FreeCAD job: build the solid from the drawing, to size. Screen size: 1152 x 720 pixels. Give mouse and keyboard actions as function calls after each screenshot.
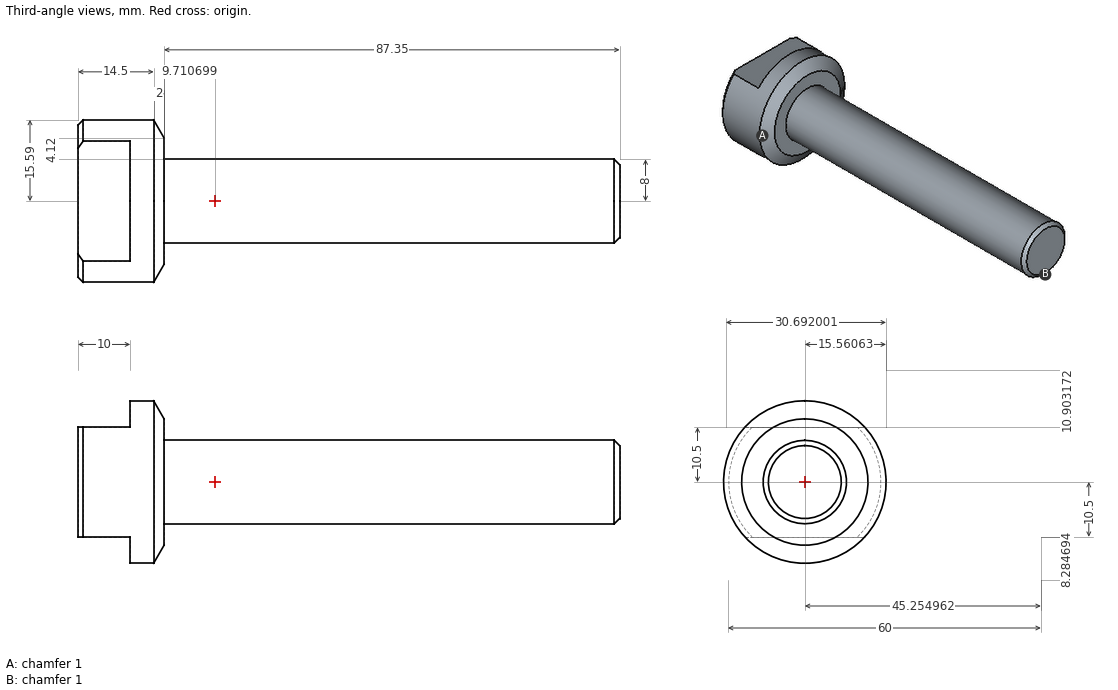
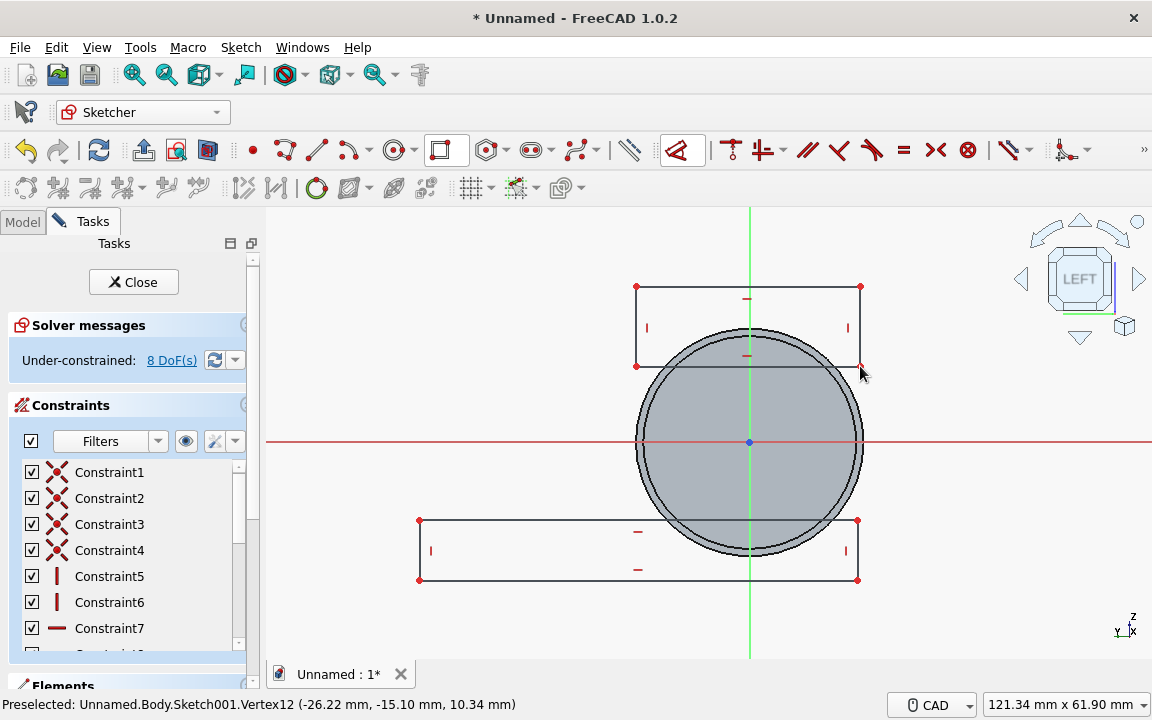
click(551, 581)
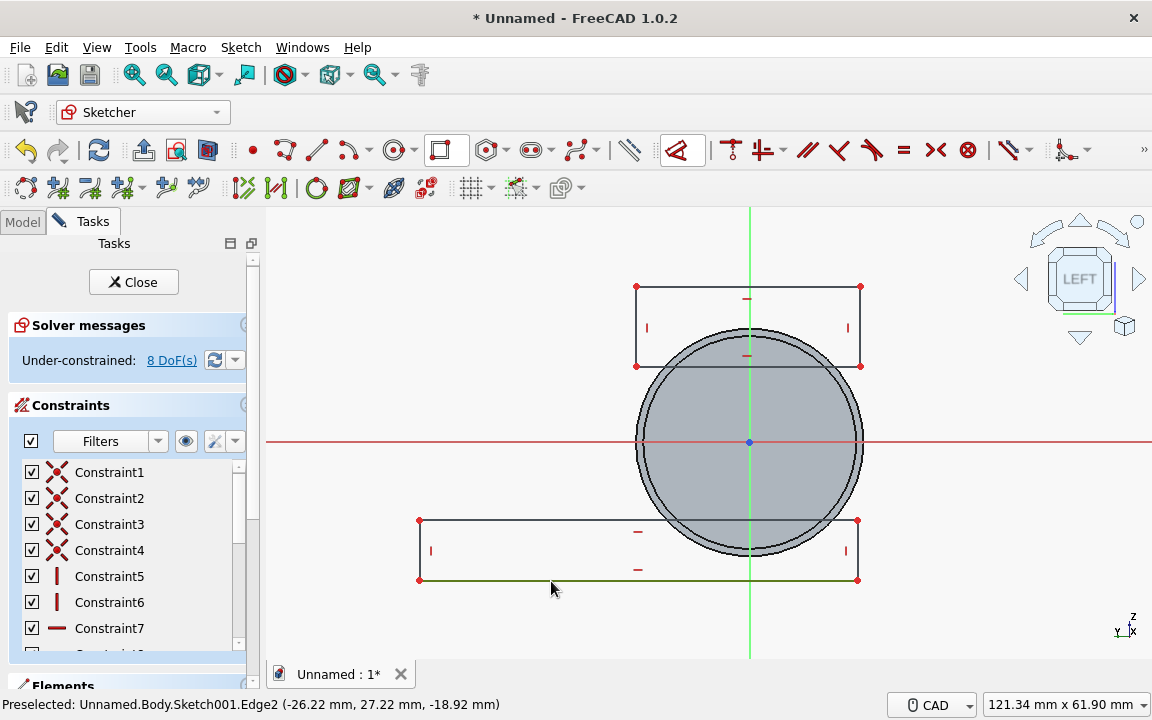
click(700, 150)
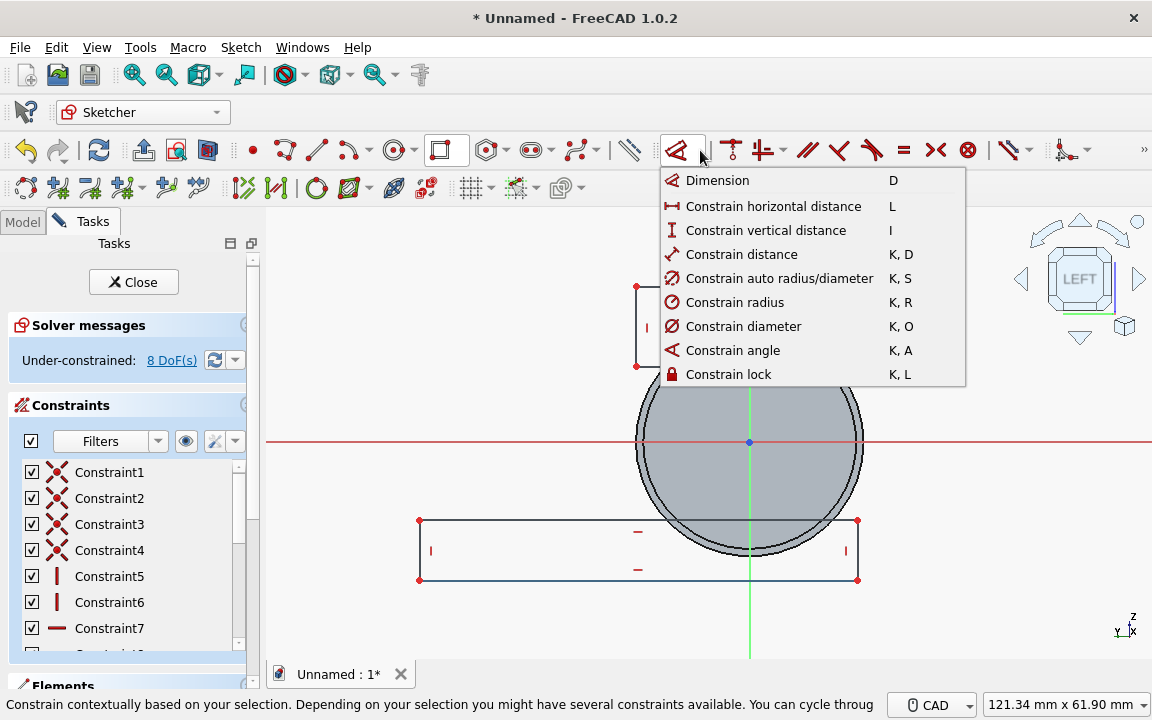
click(813, 206)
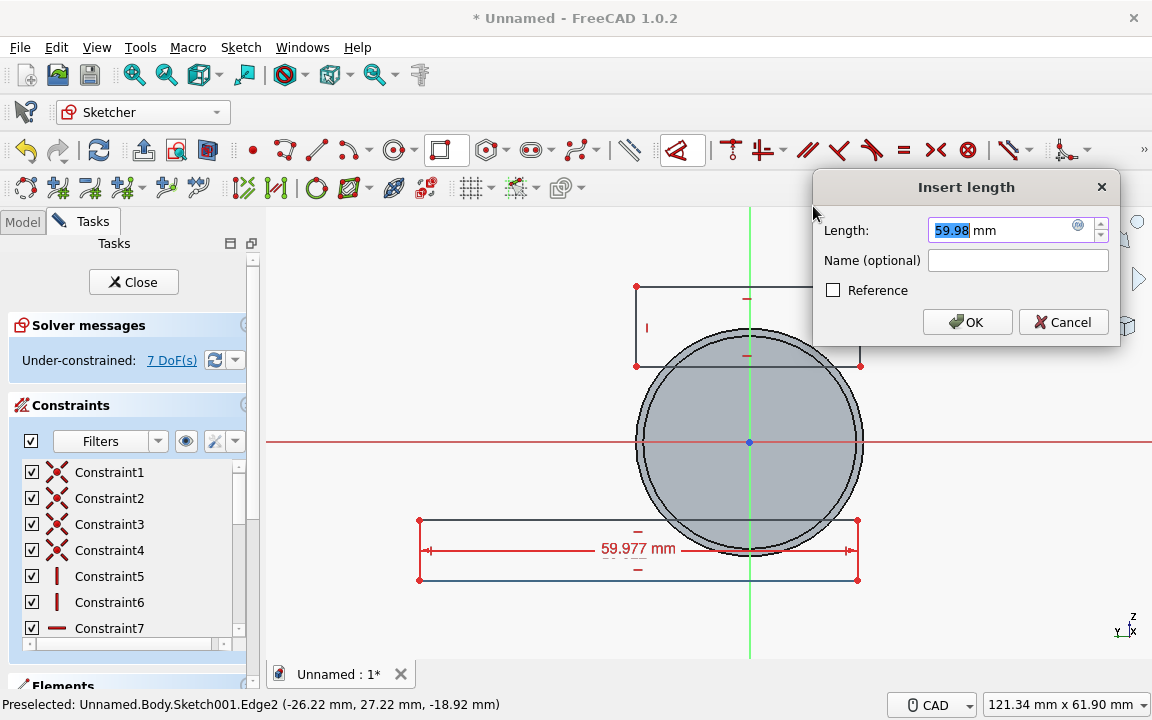
text(60)
key(Return)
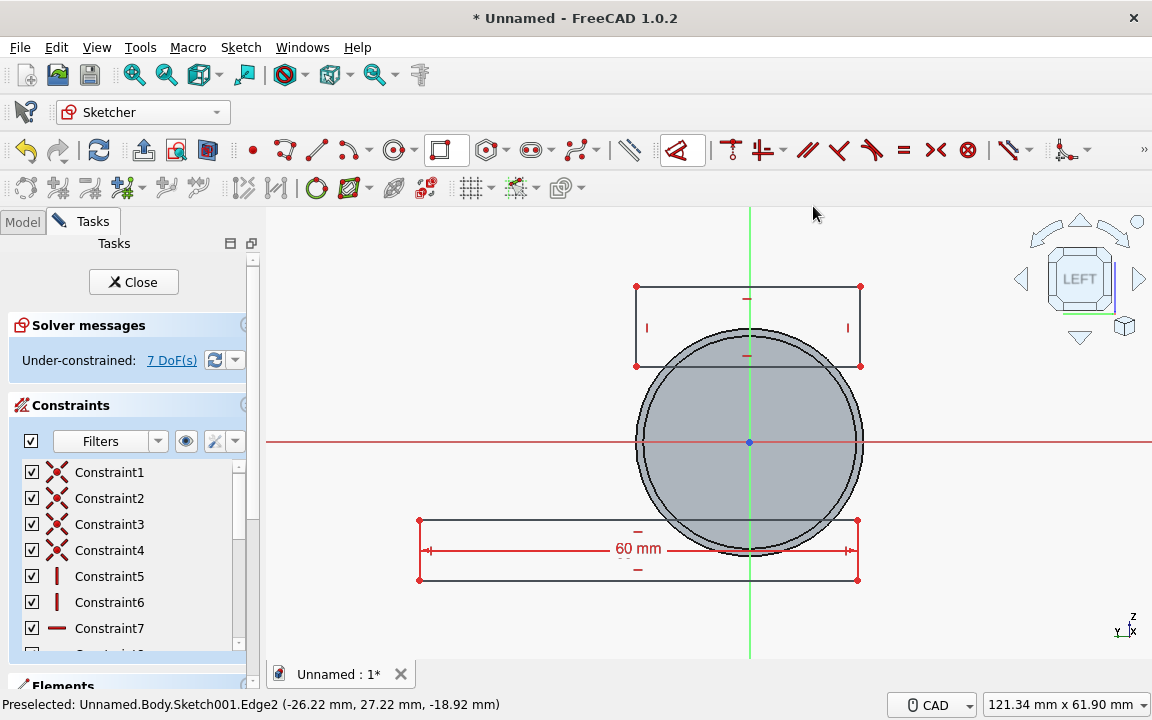
click(420, 520)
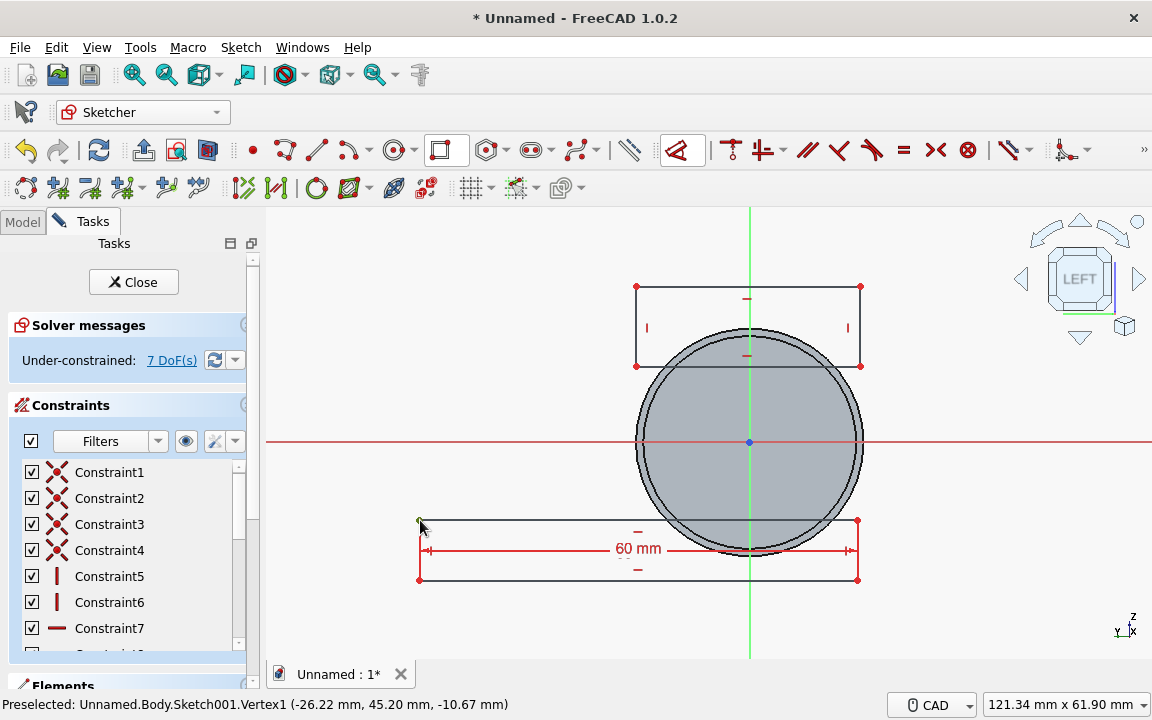
key(i)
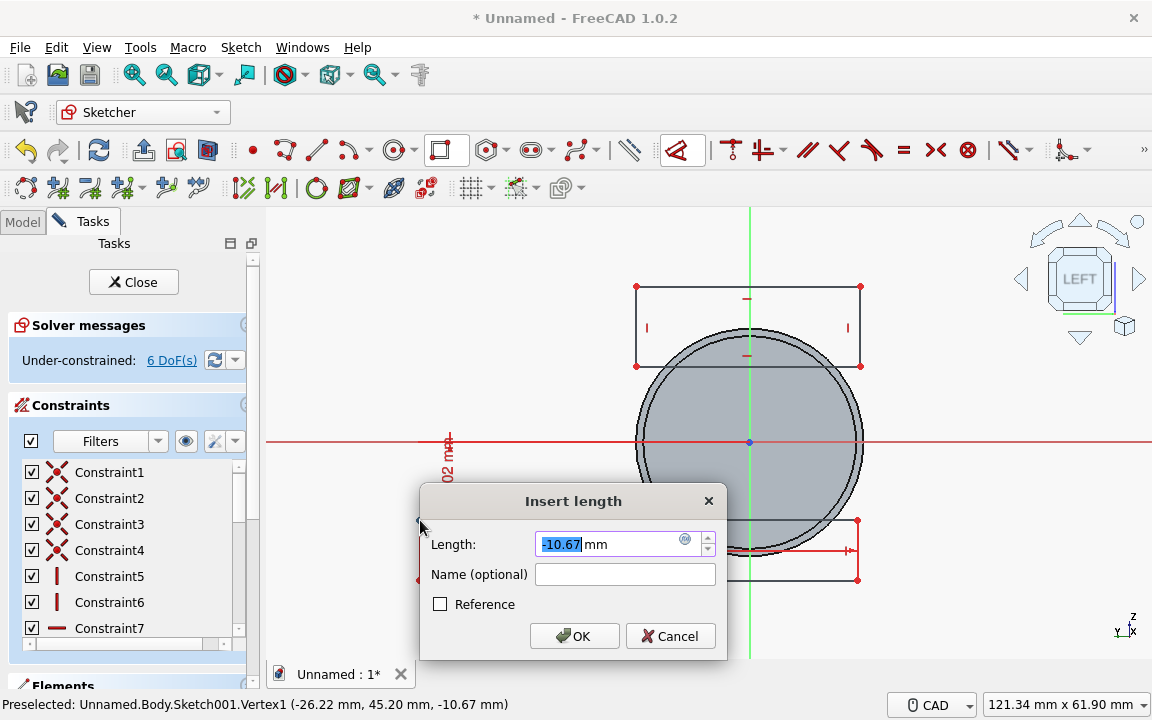
text(-10.5)
key(Return)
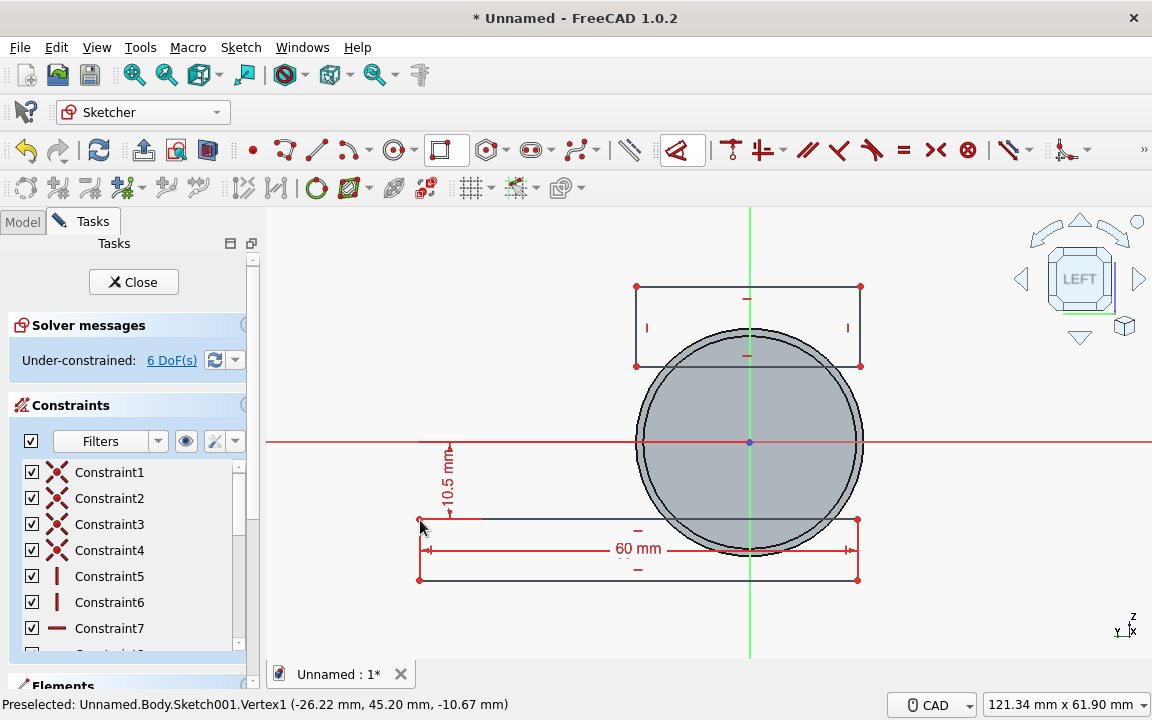
click(636, 367)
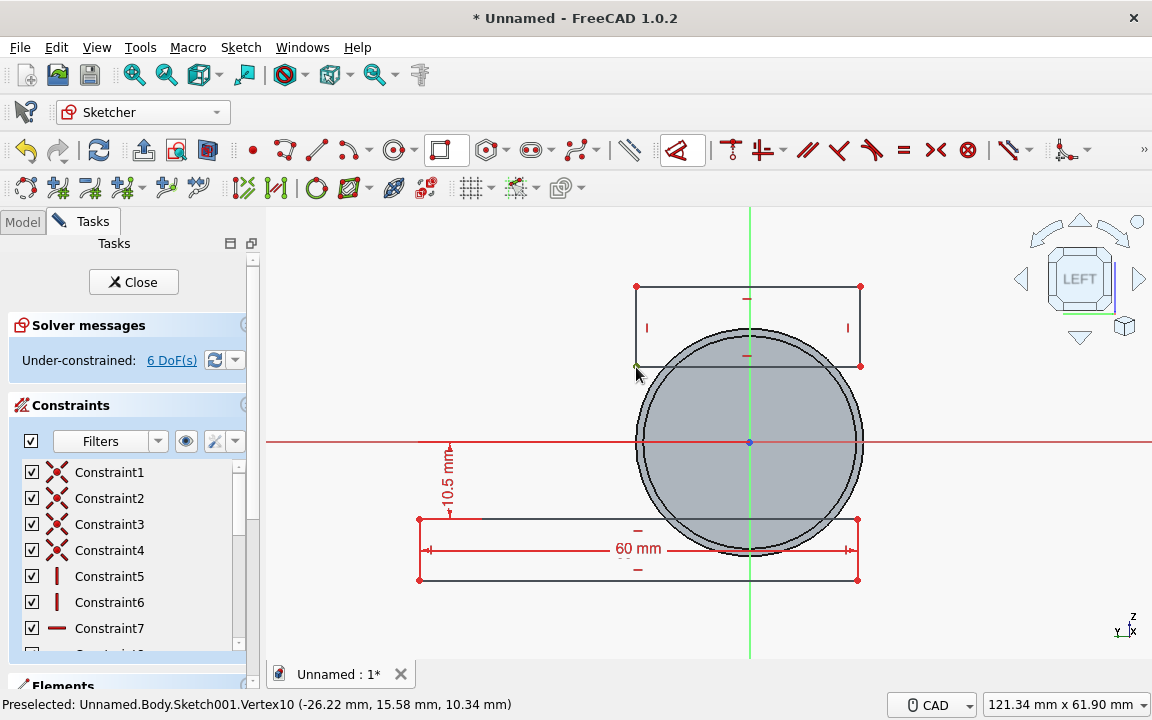
key(i)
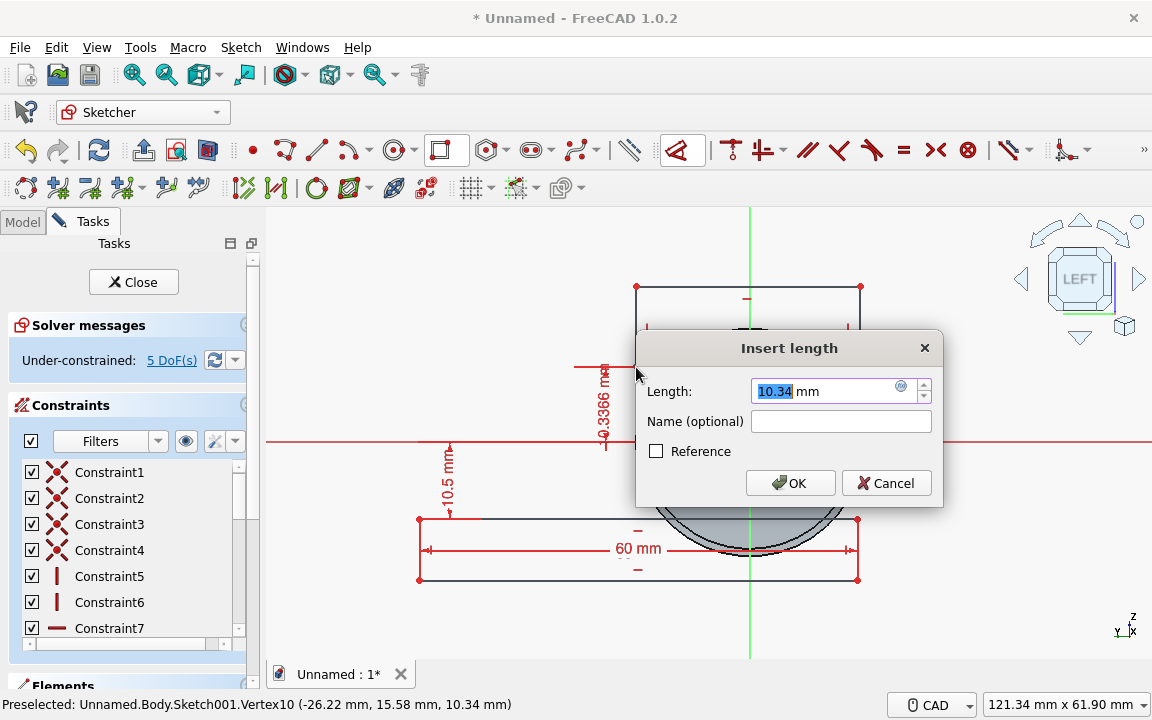
text(10.5)
key(Return)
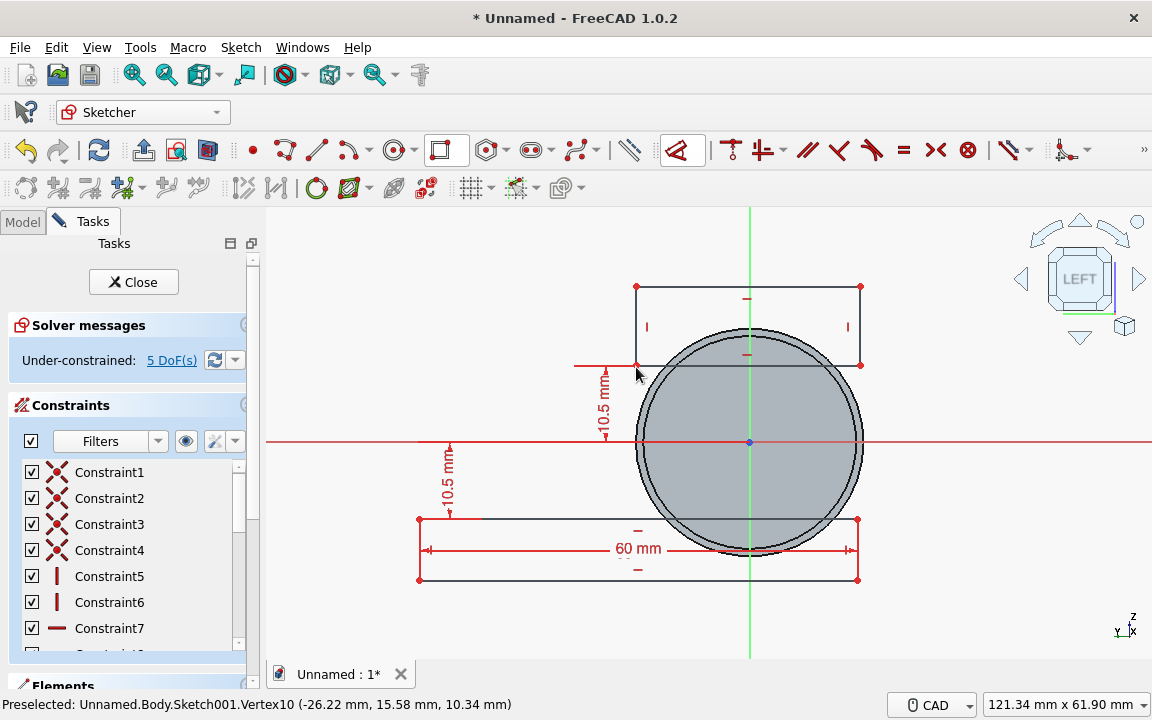
click(420, 538)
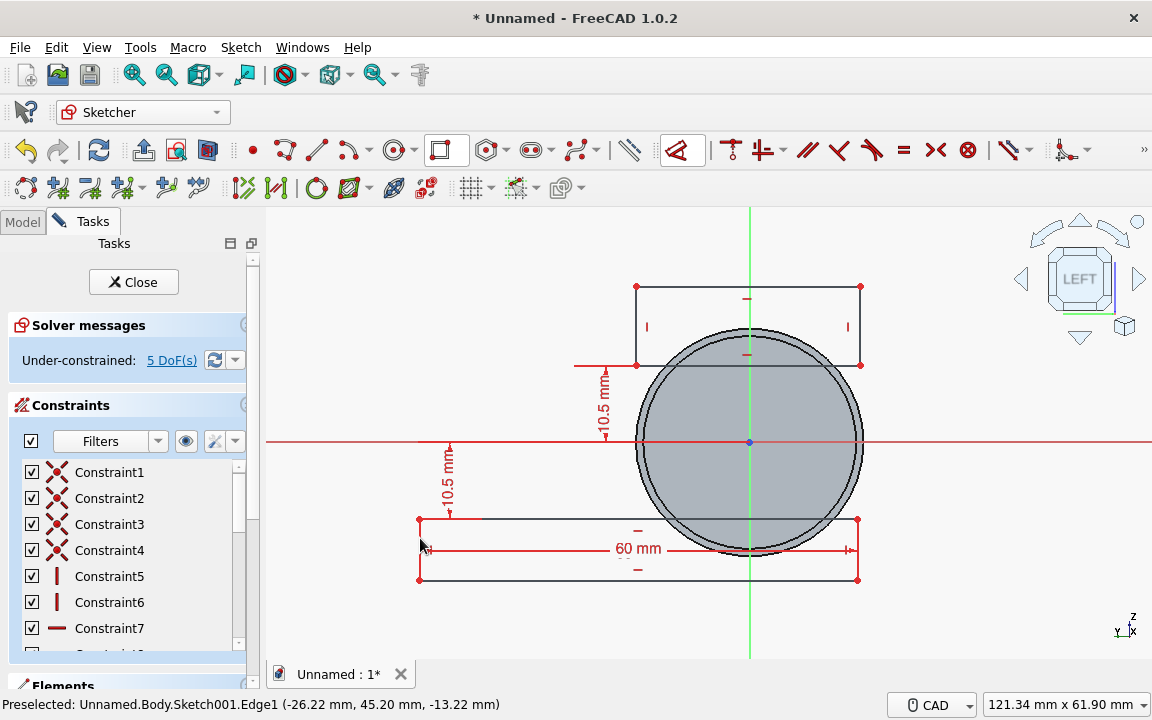
click(700, 150)